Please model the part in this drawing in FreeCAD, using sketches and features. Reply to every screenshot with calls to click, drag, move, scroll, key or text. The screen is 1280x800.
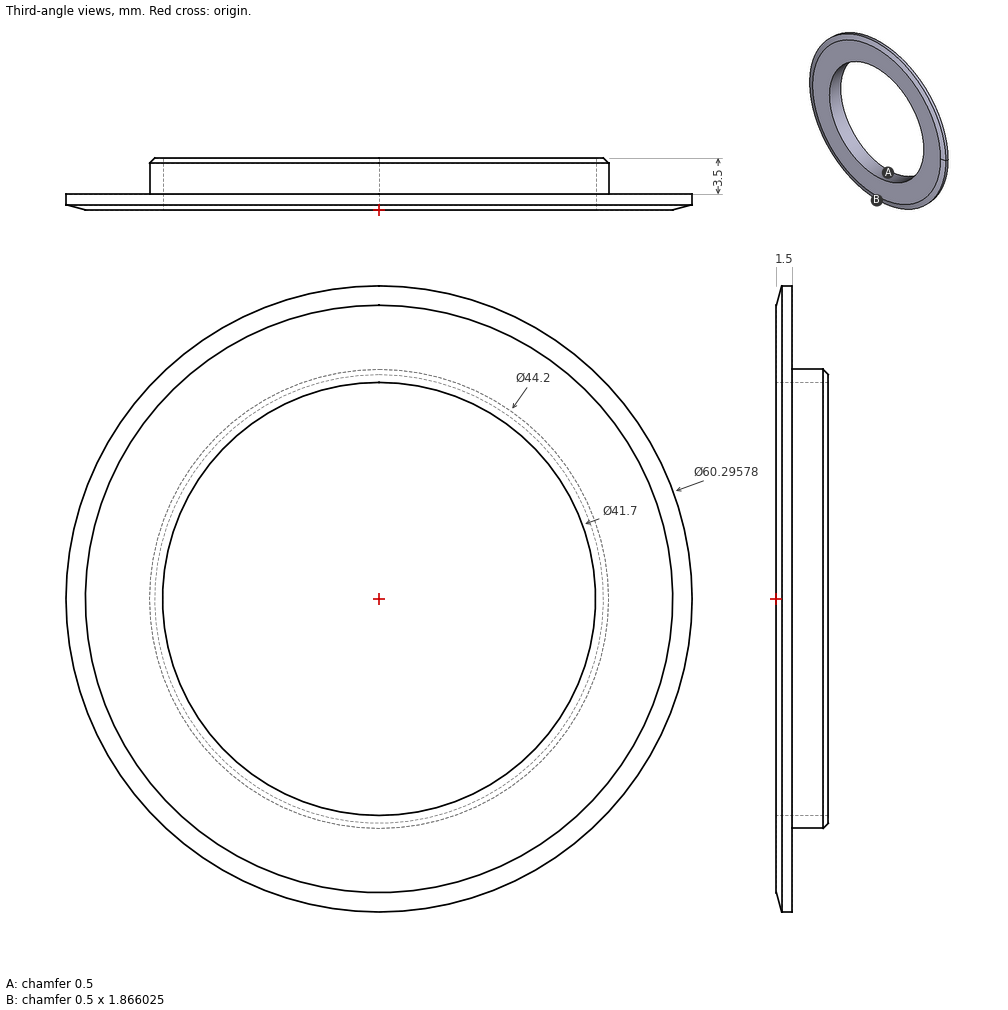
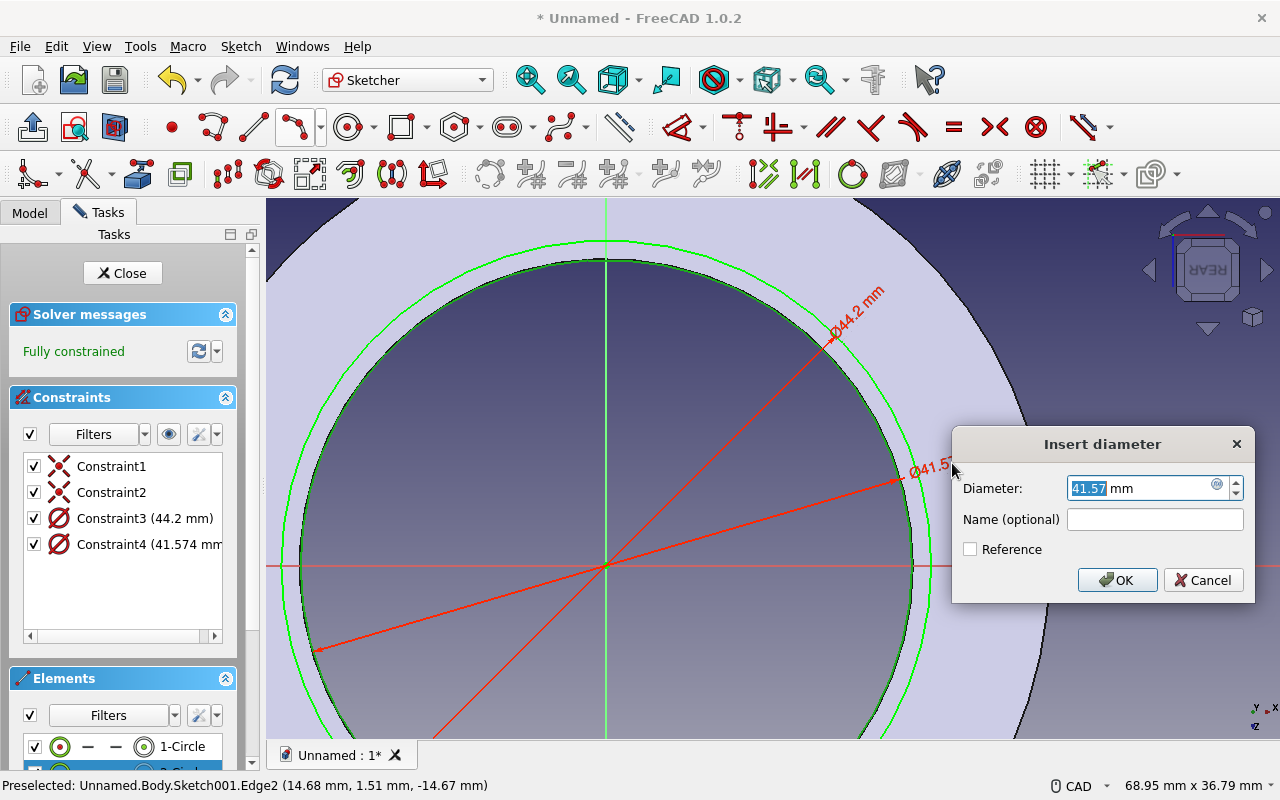
text(41.7)
key(Return)
key(Escape)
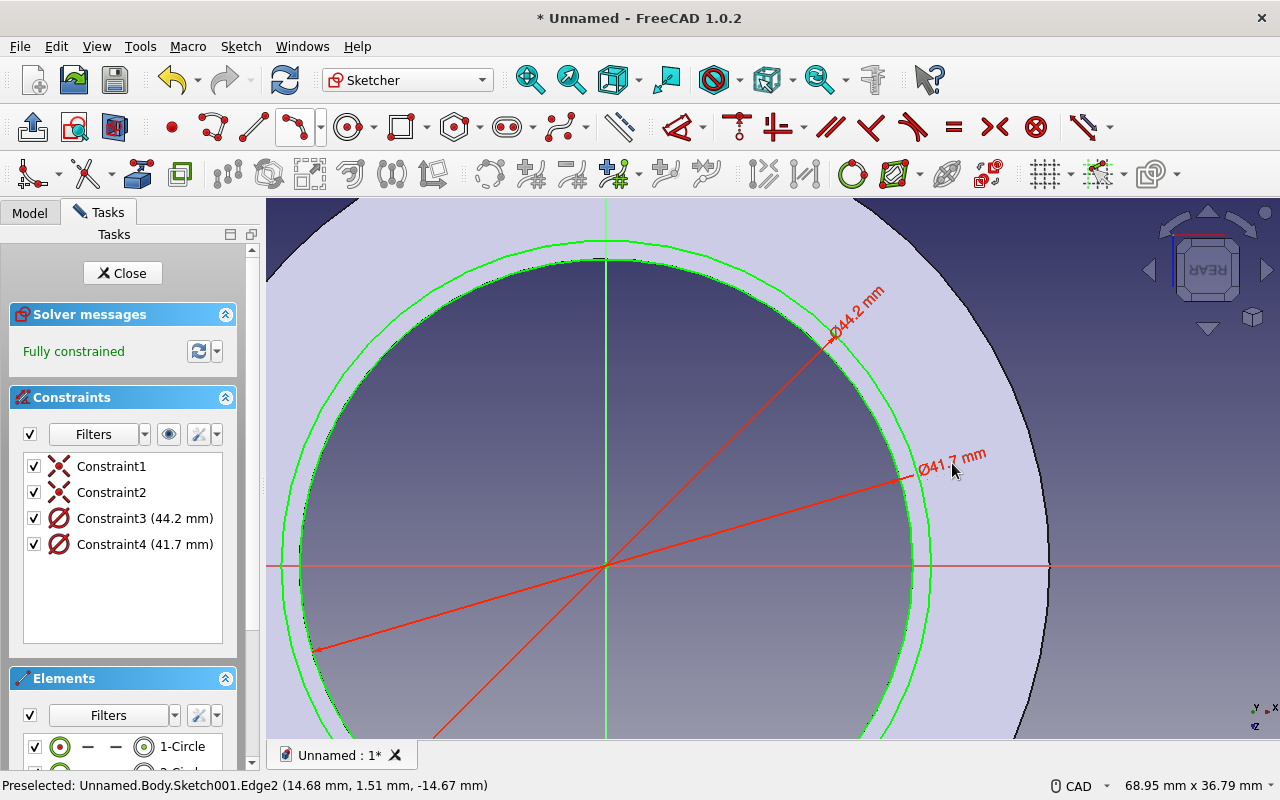
click(123, 273)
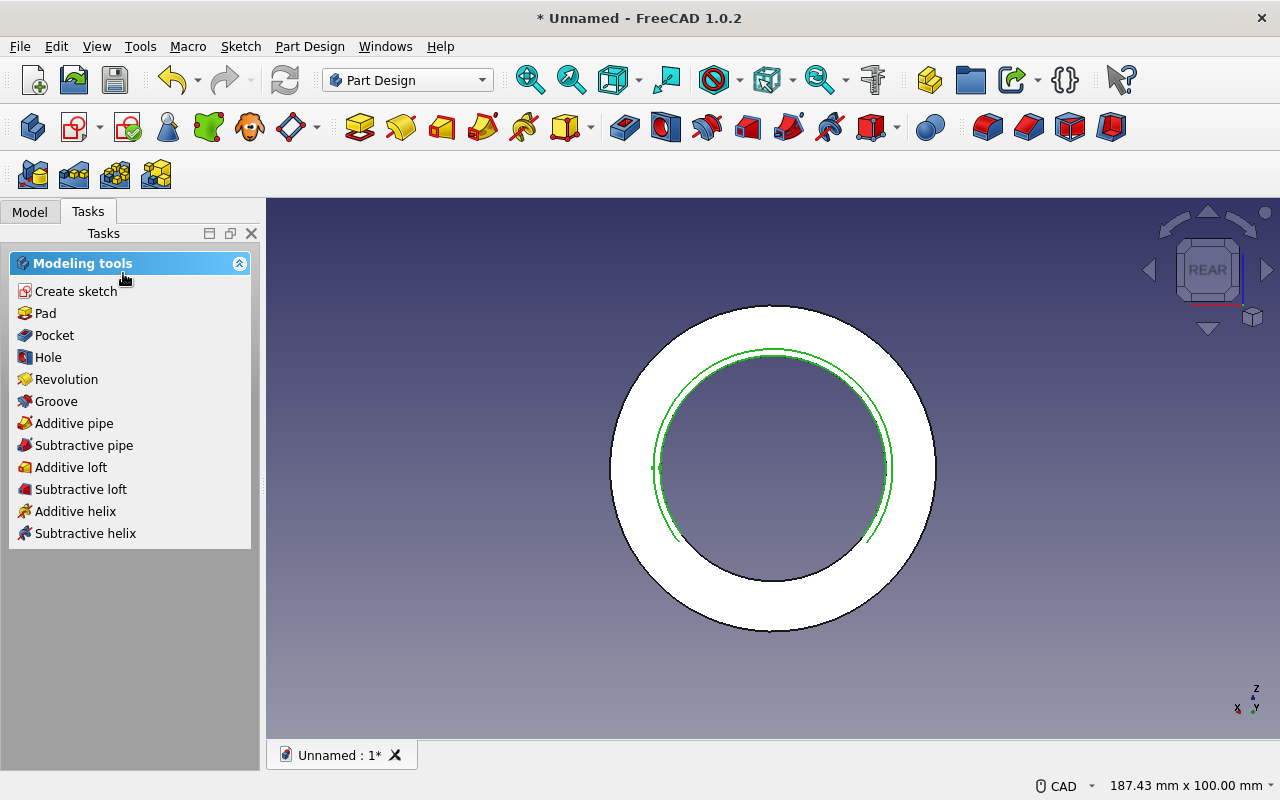
click(360, 128)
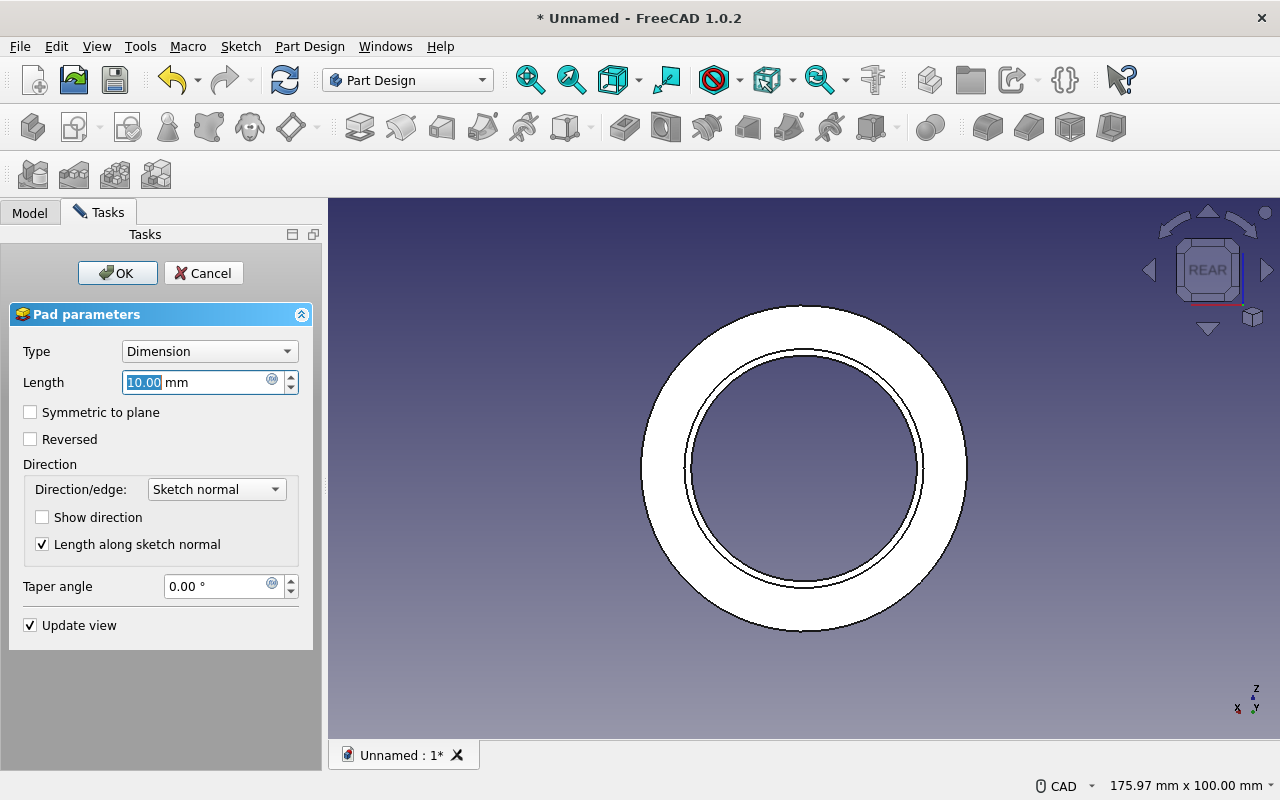
text(3.5)
key(Tab)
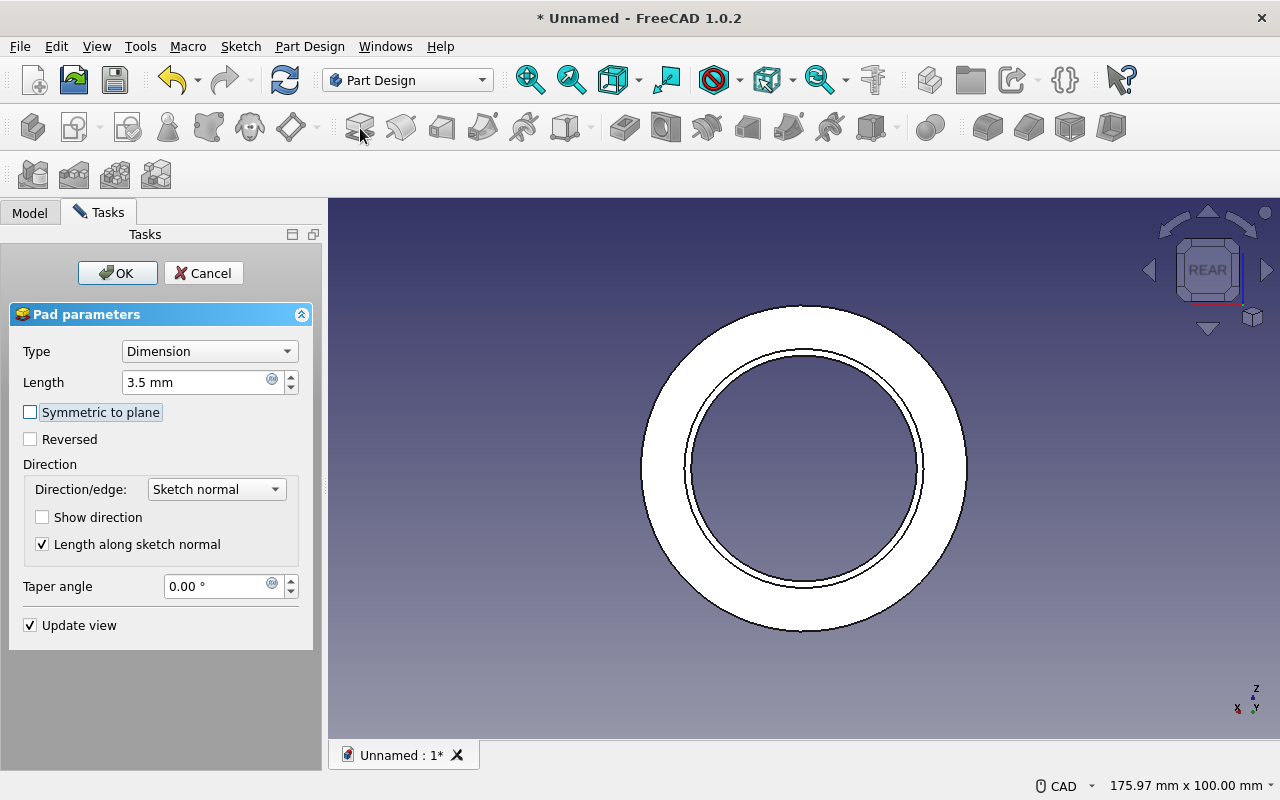
click(118, 273)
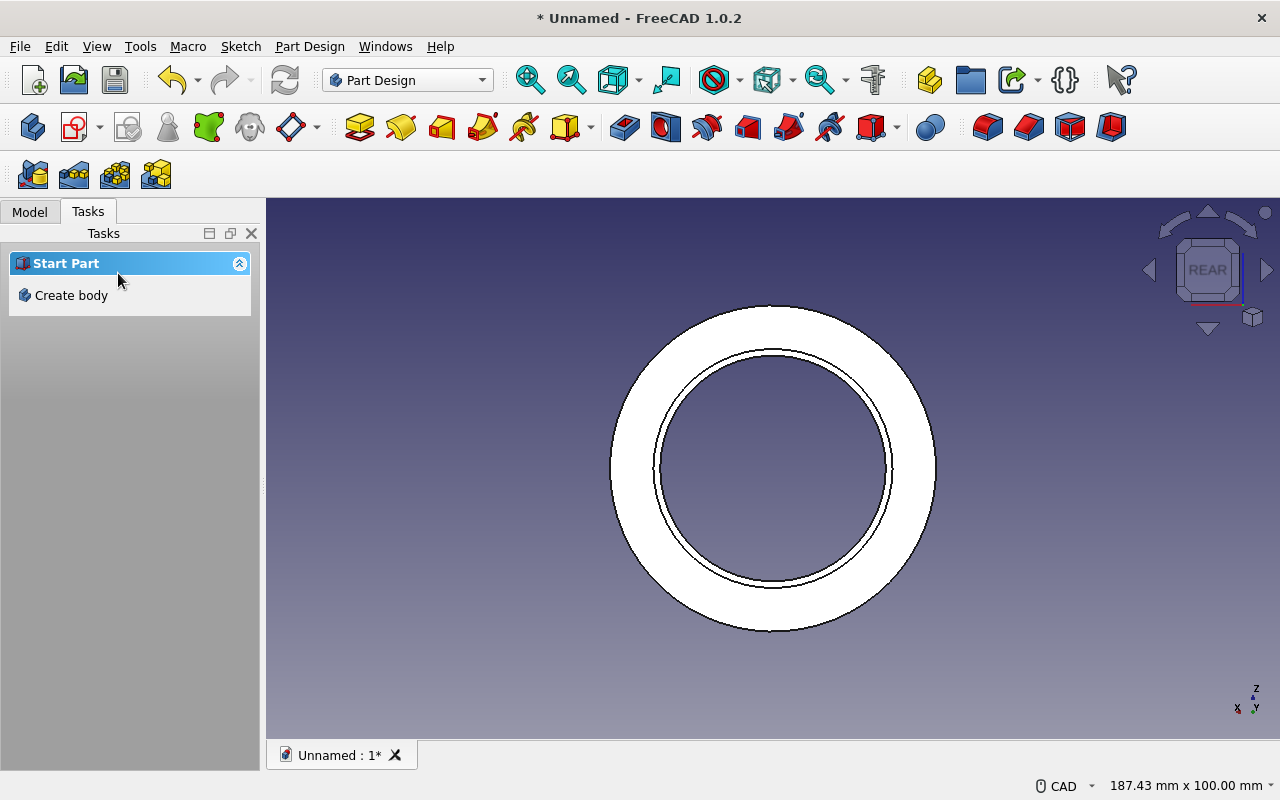
click(893, 467)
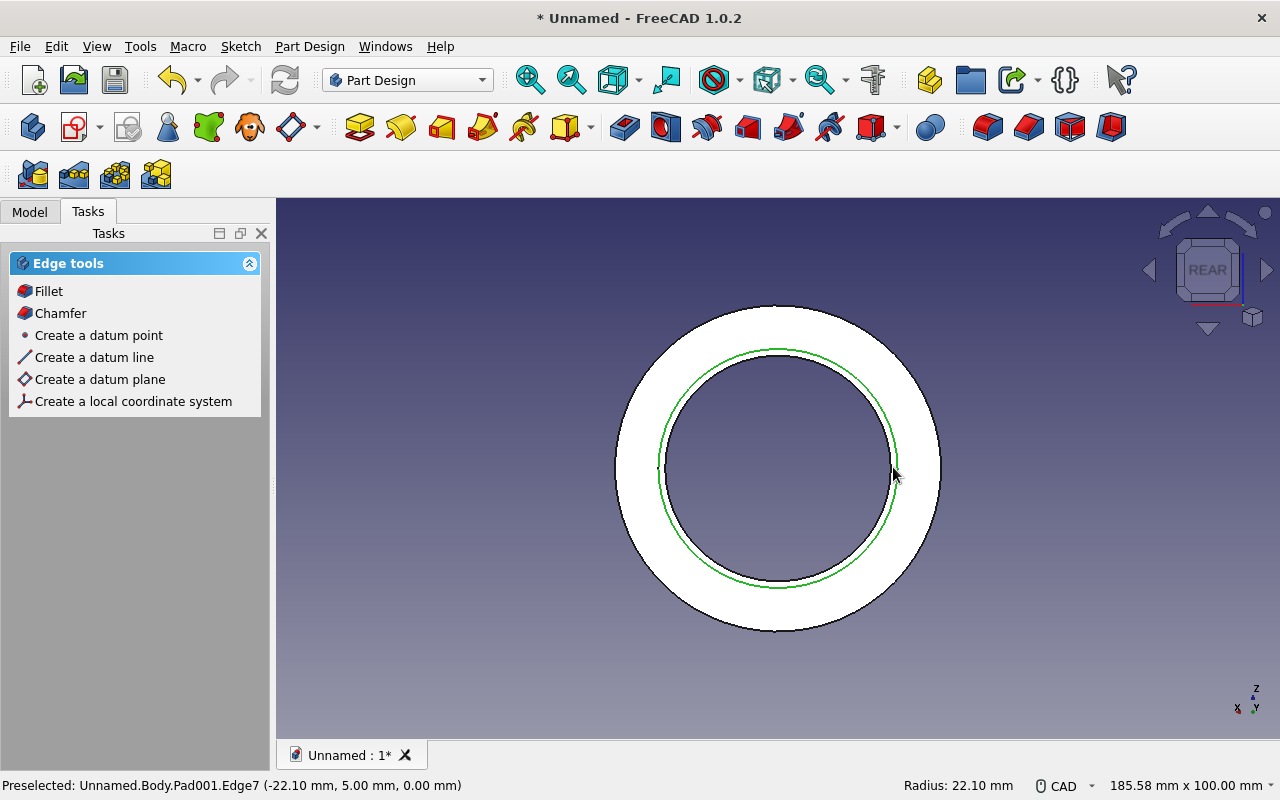
click(1029, 128)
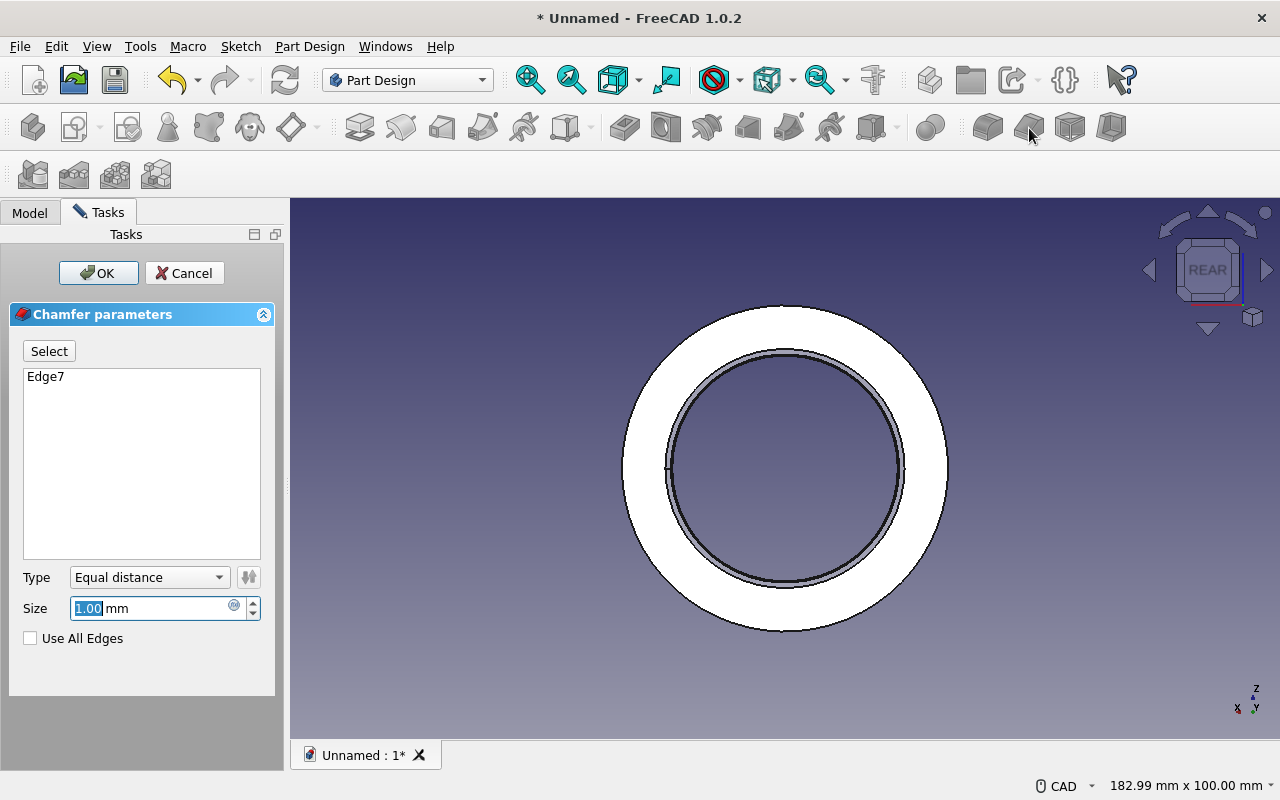
text(0.5)
key(Tab)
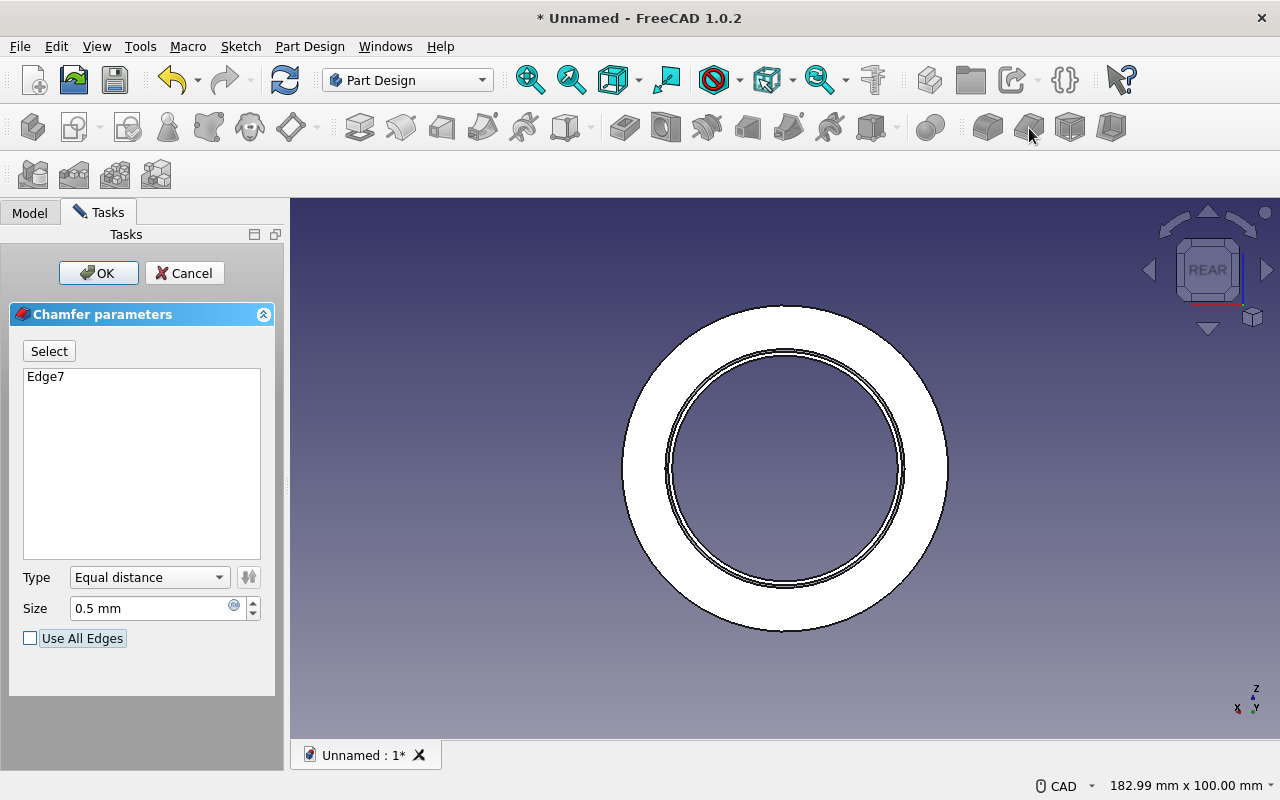
click(99, 273)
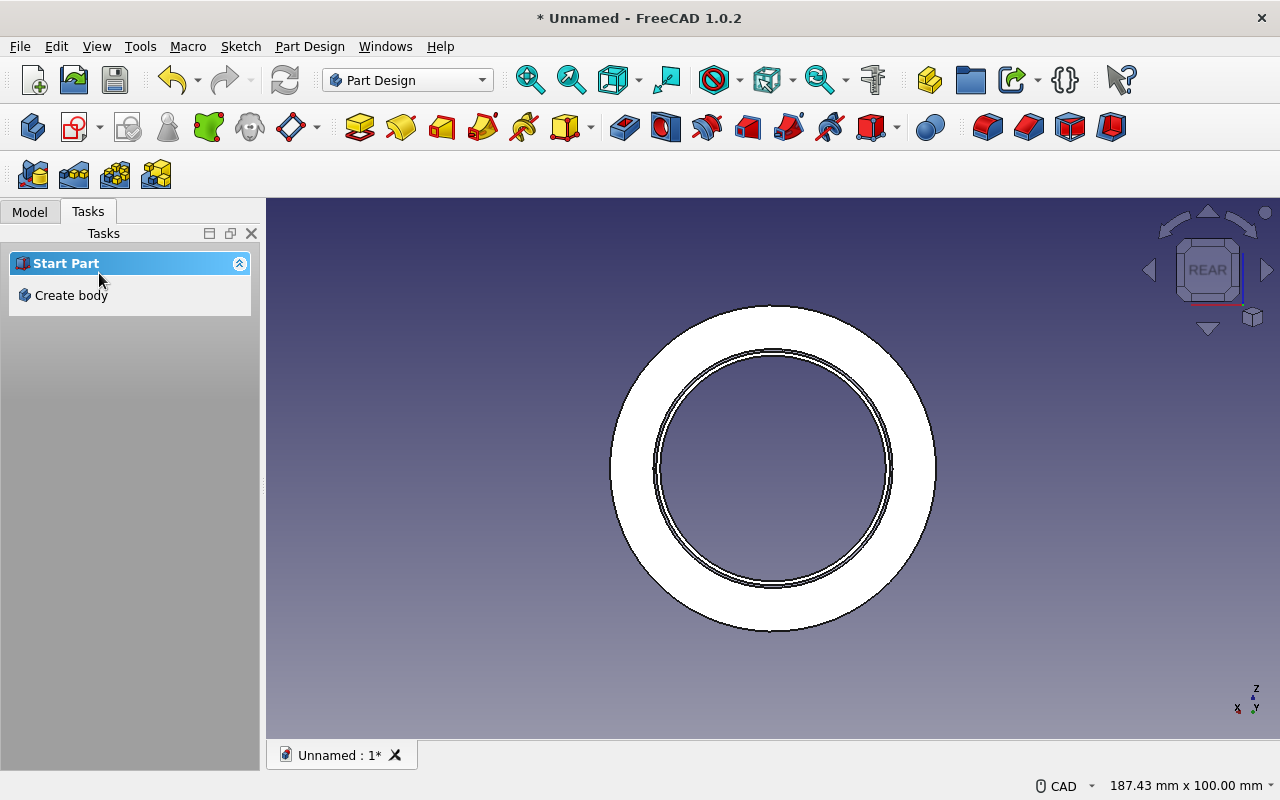
key(0)